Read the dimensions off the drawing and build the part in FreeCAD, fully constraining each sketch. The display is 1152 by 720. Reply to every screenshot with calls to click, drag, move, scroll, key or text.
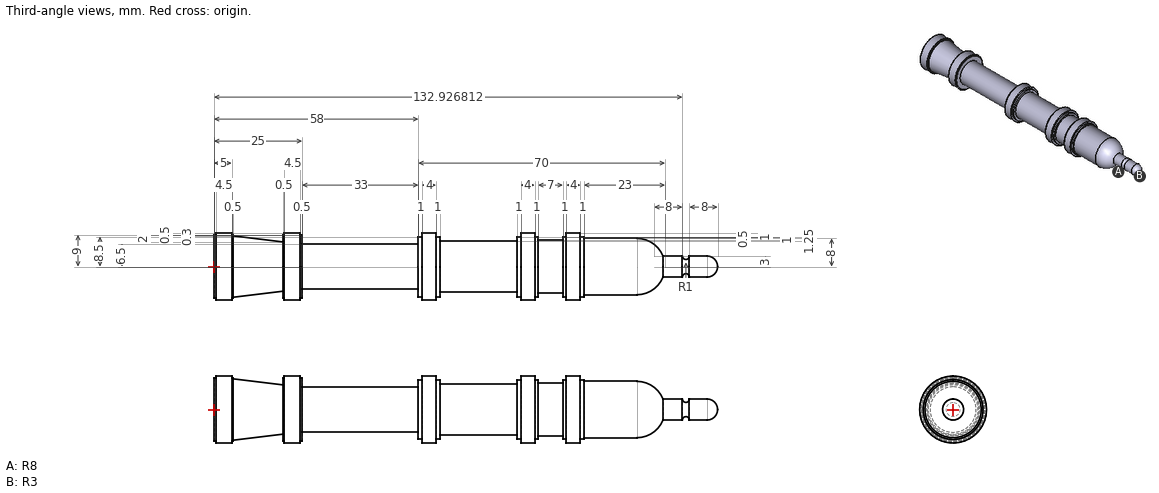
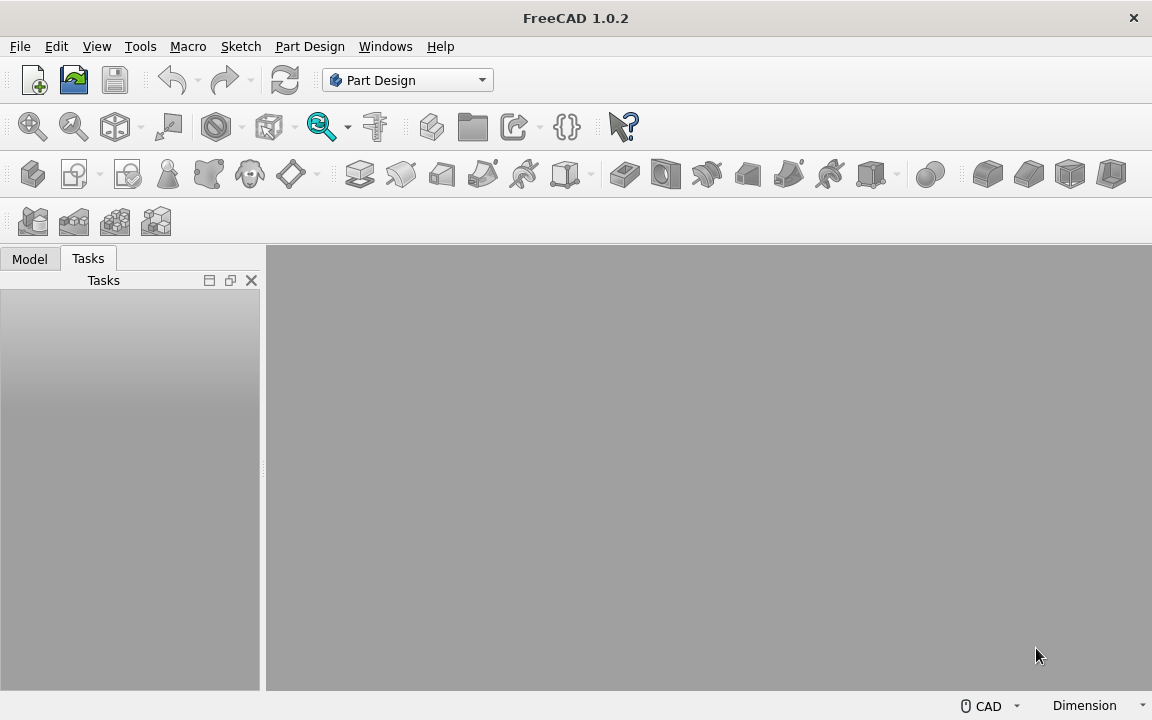
click(33, 80)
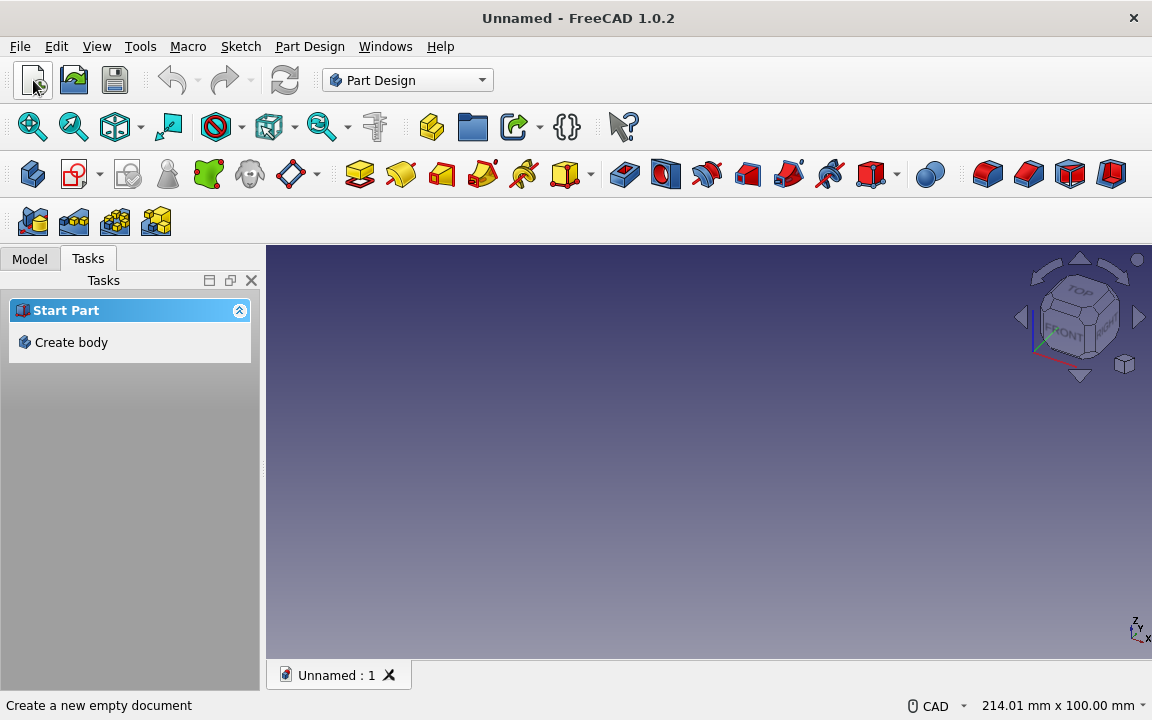
click(74, 174)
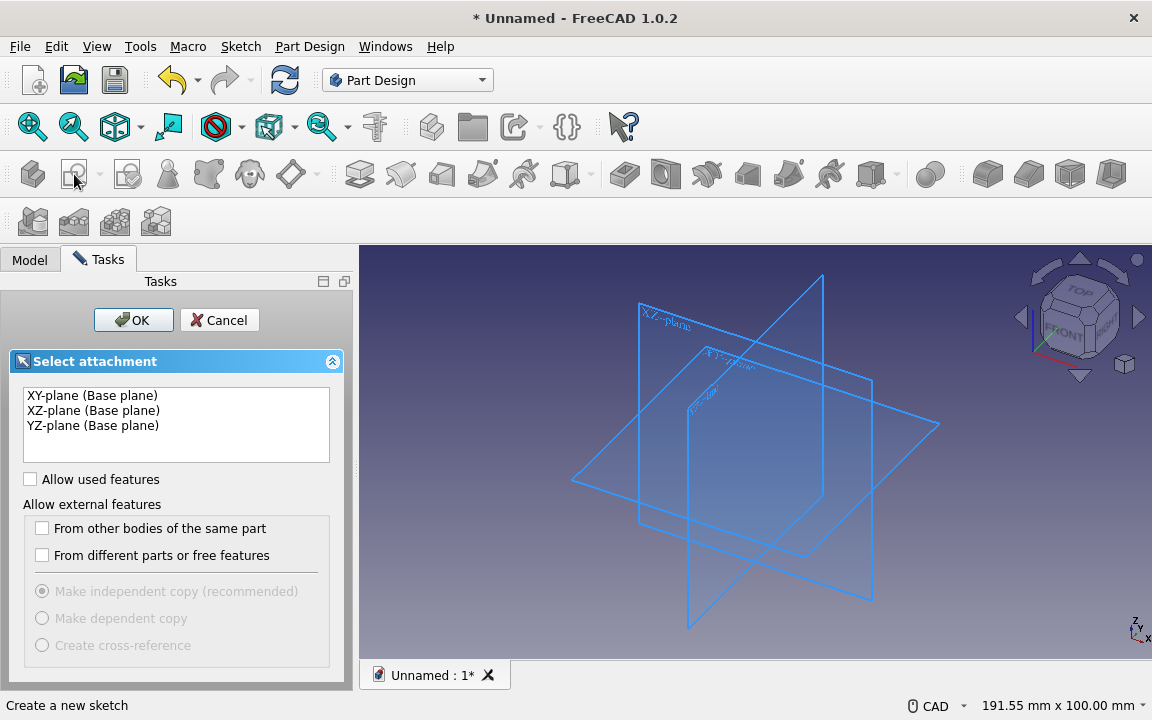
click(84, 396)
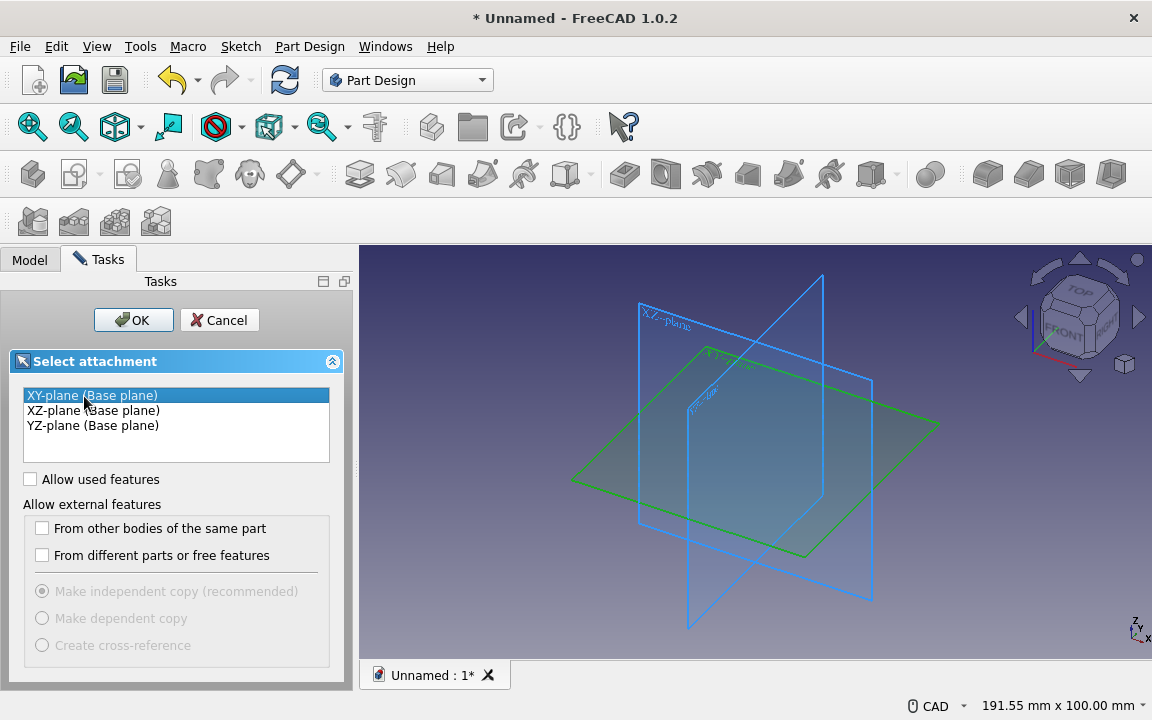
click(134, 320)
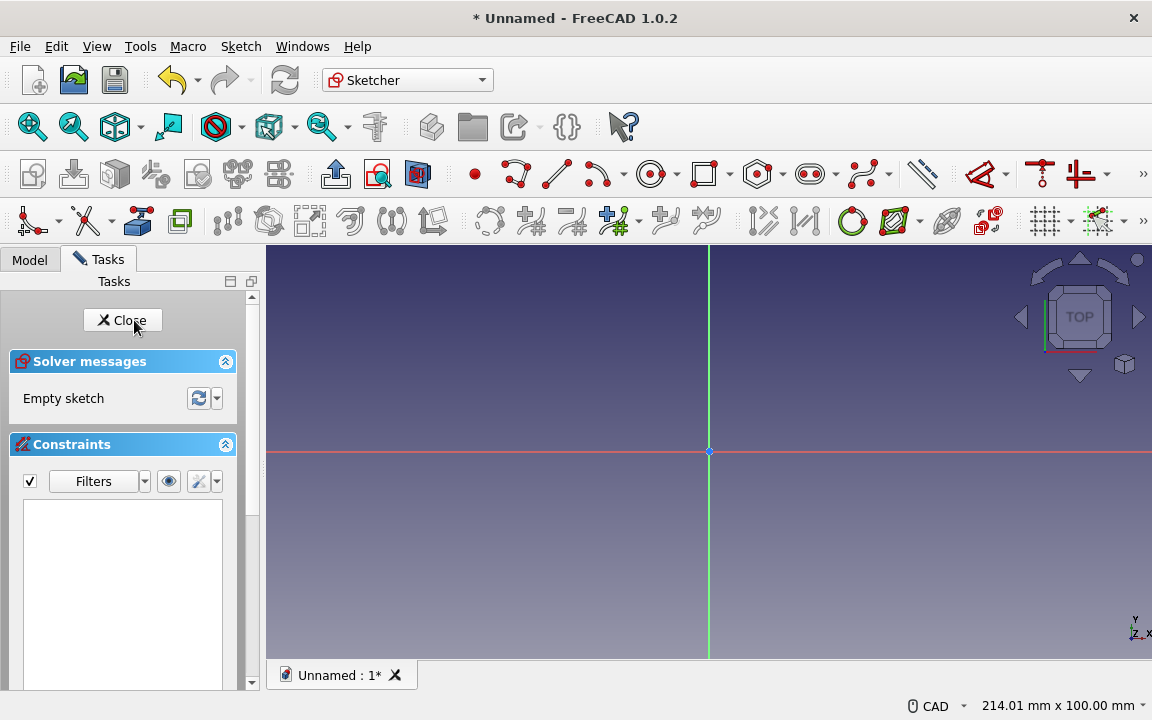
scroll(791, 427, up, 8)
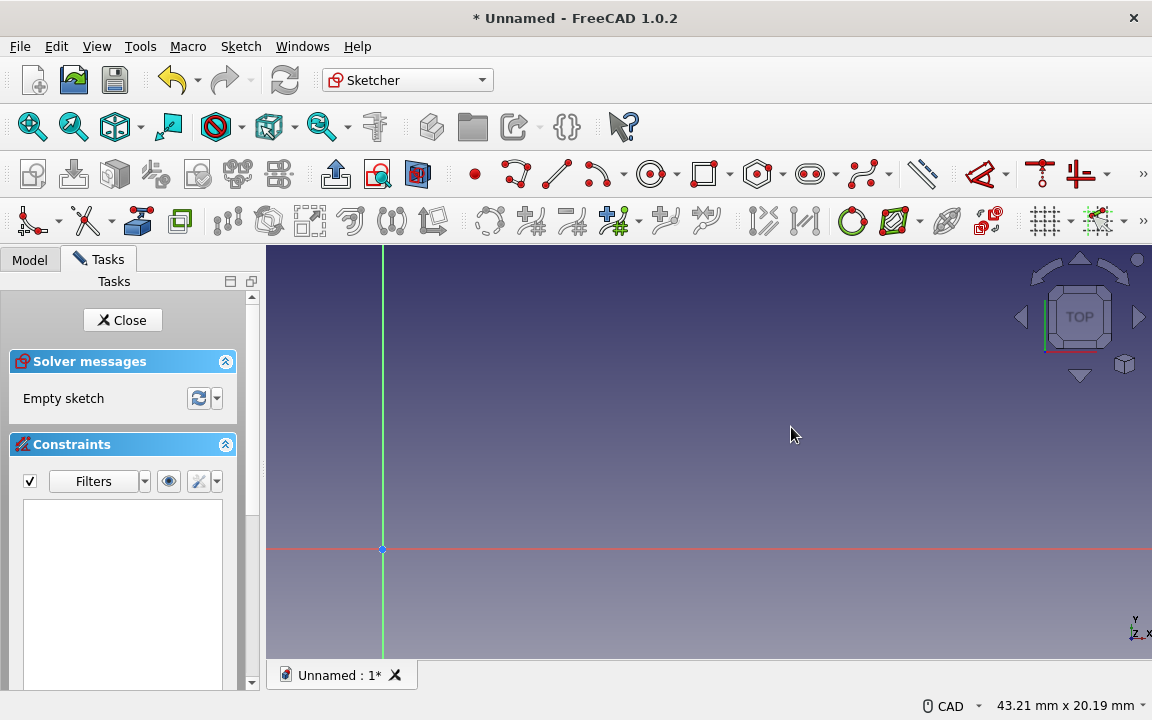
click(516, 174)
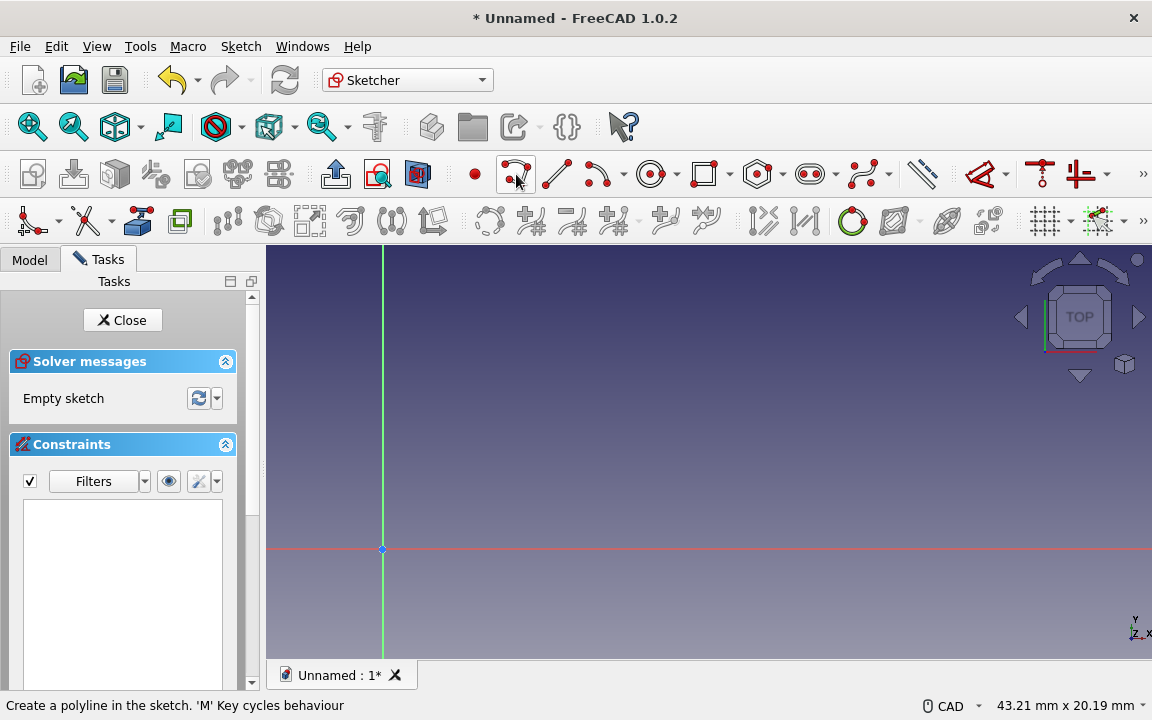
click(383, 549)
click(895, 540)
click(895, 365)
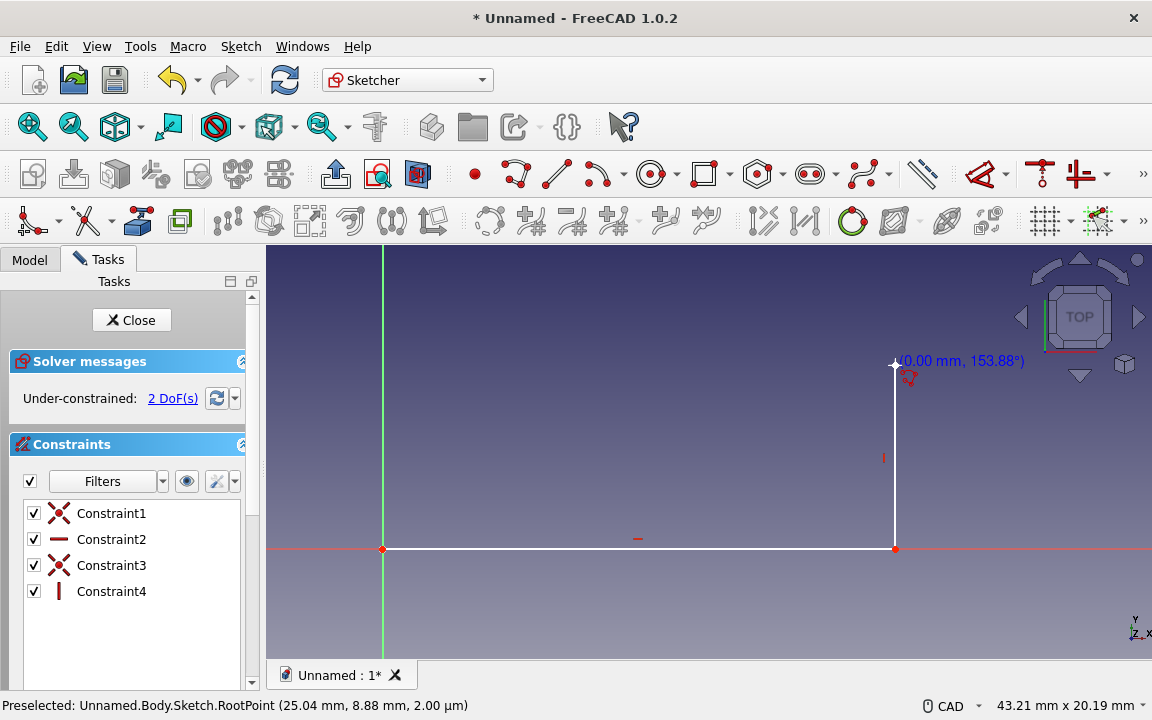
scroll(885, 365, up, 3)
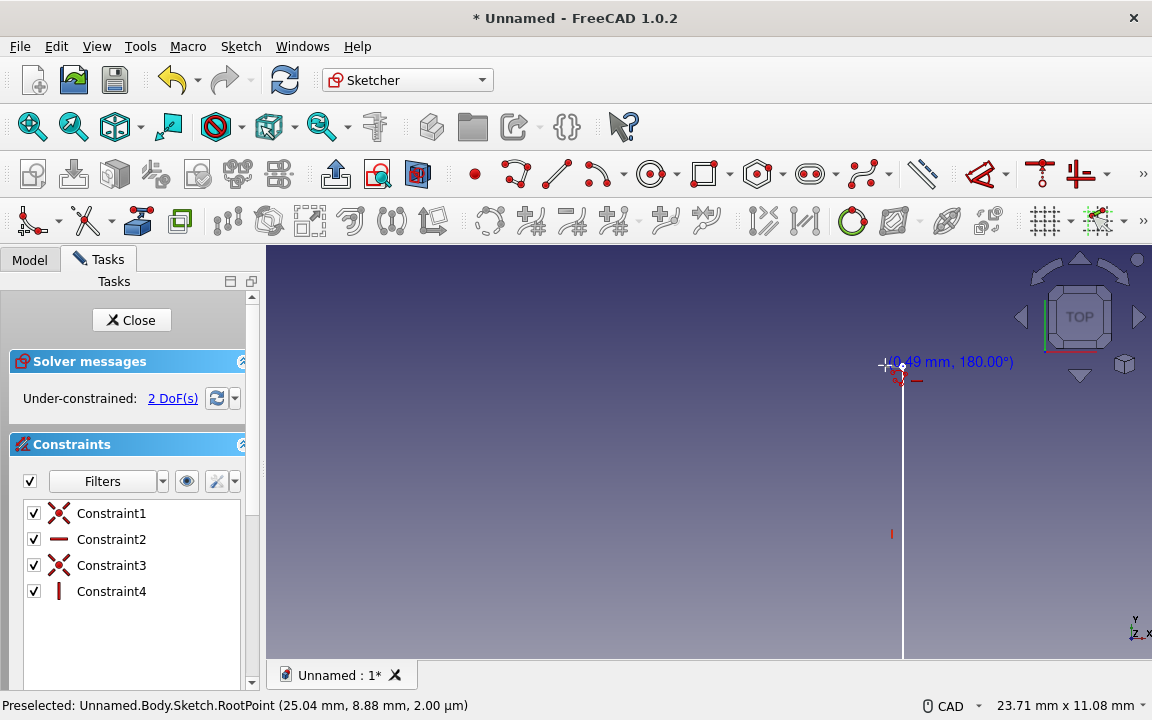
click(884, 365)
click(884, 345)
click(716, 345)
click(716, 364)
click(697, 364)
click(697, 439)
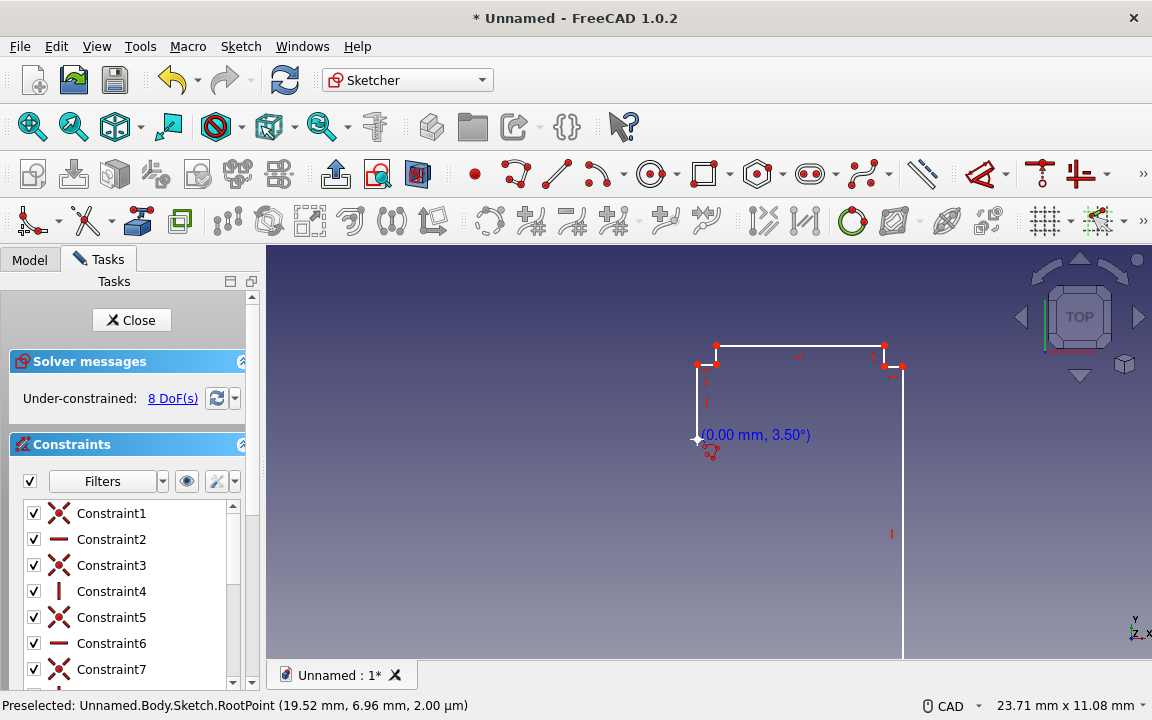
scroll(889, 366, down, 3)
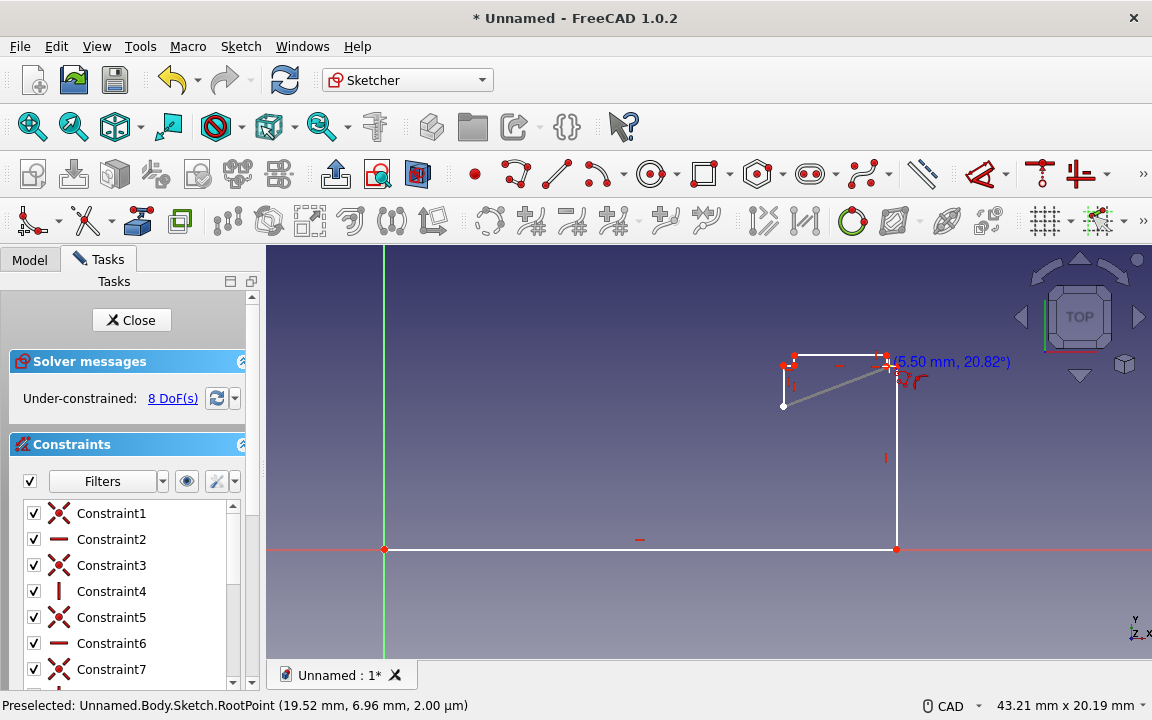
click(497, 371)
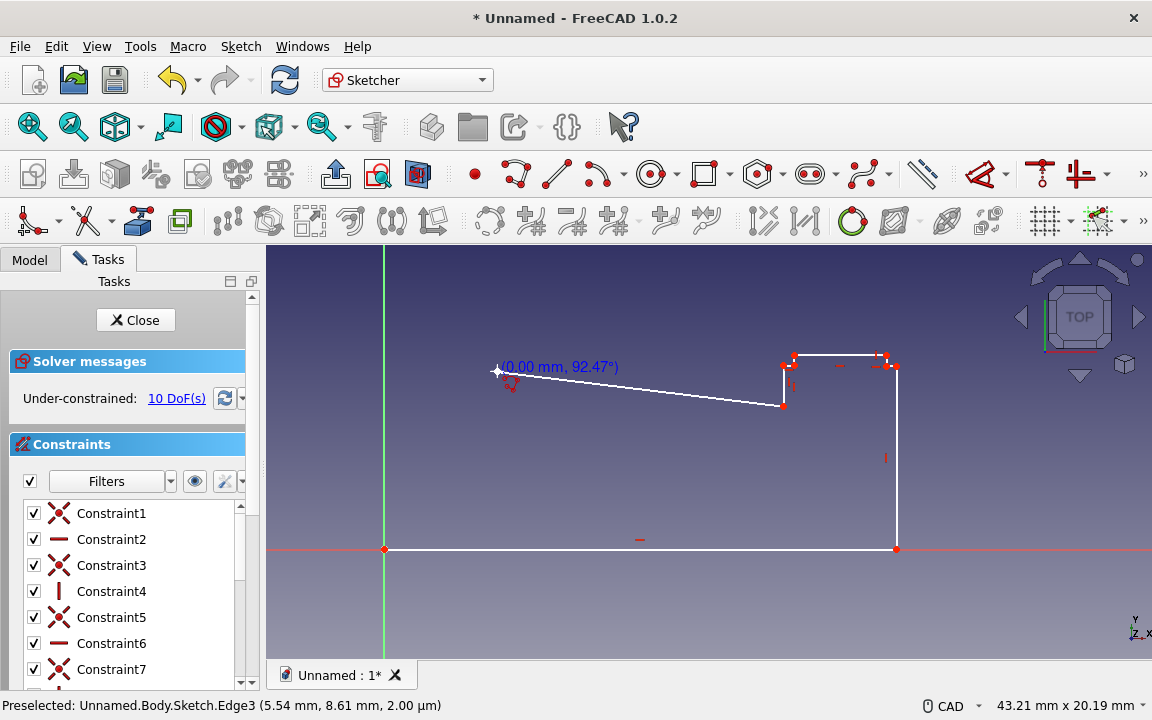
scroll(497, 365, up, 5)